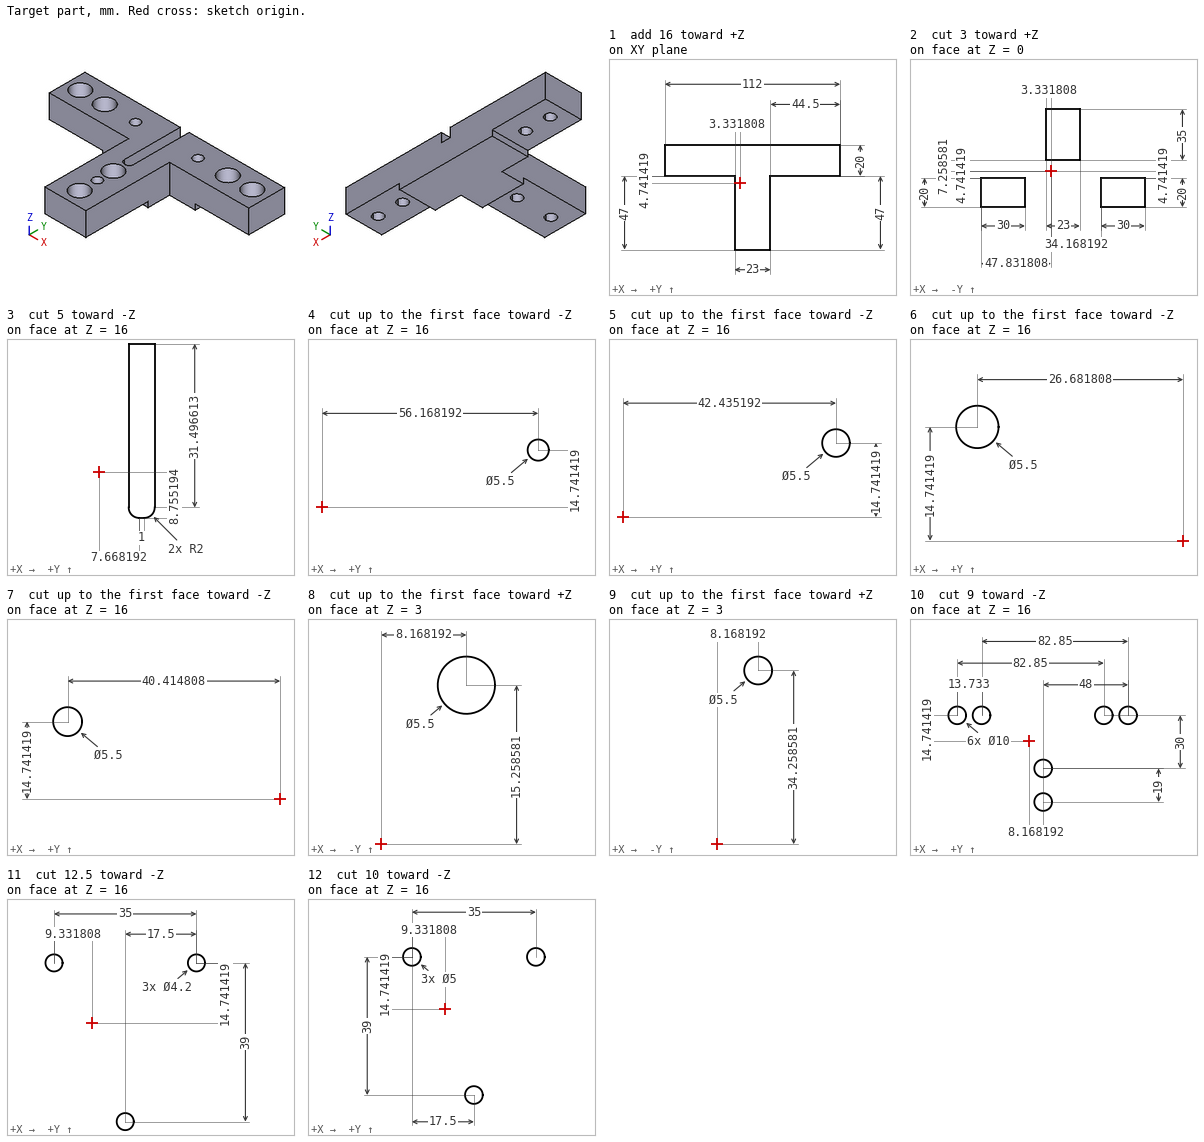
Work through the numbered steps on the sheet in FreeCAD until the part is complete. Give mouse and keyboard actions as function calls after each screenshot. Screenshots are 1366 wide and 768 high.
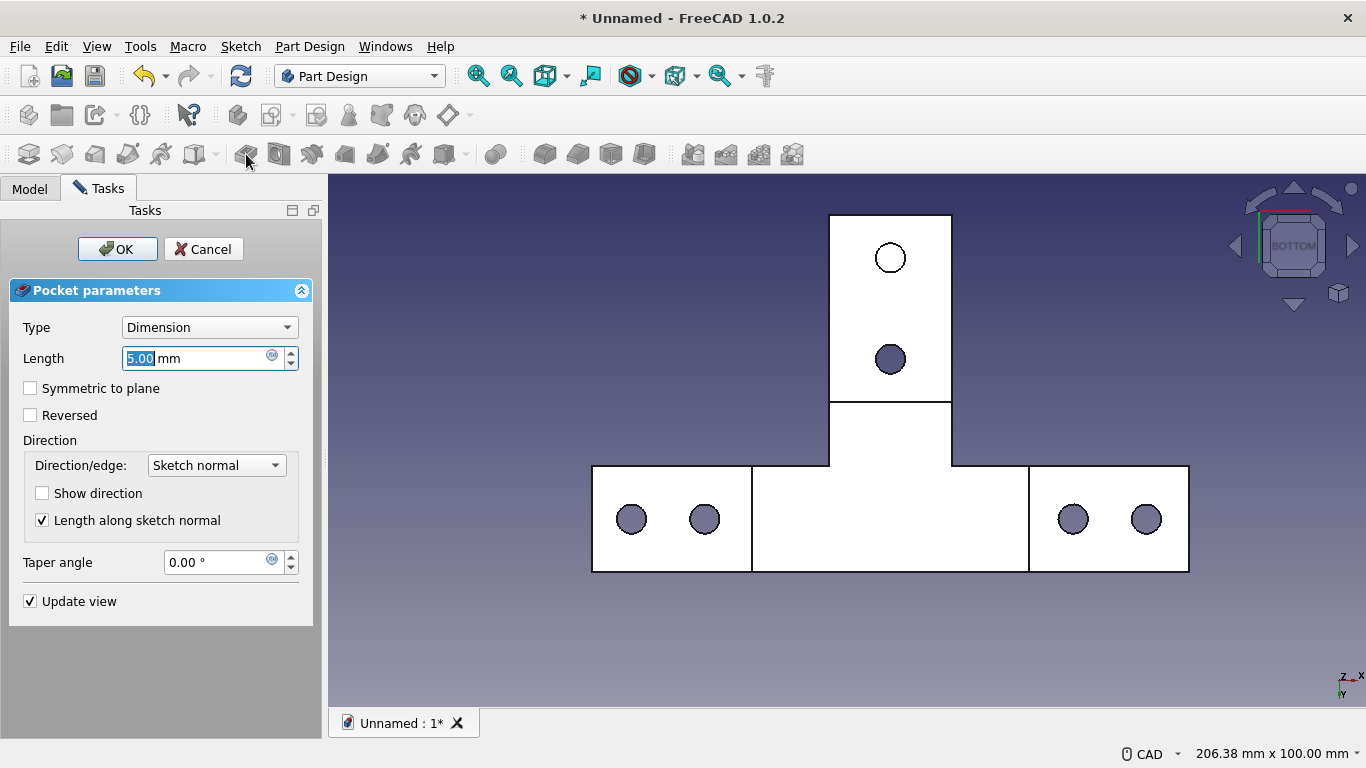
click(210, 328)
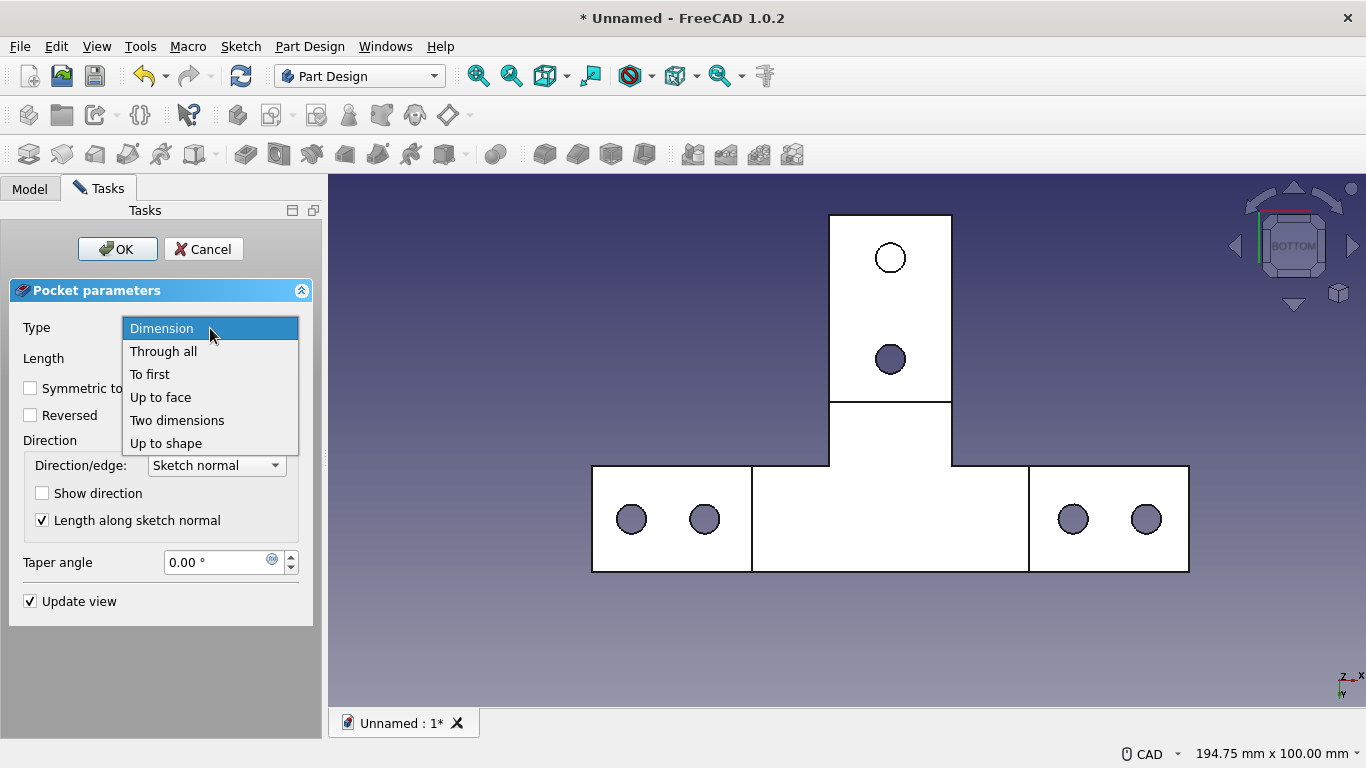
click(208, 374)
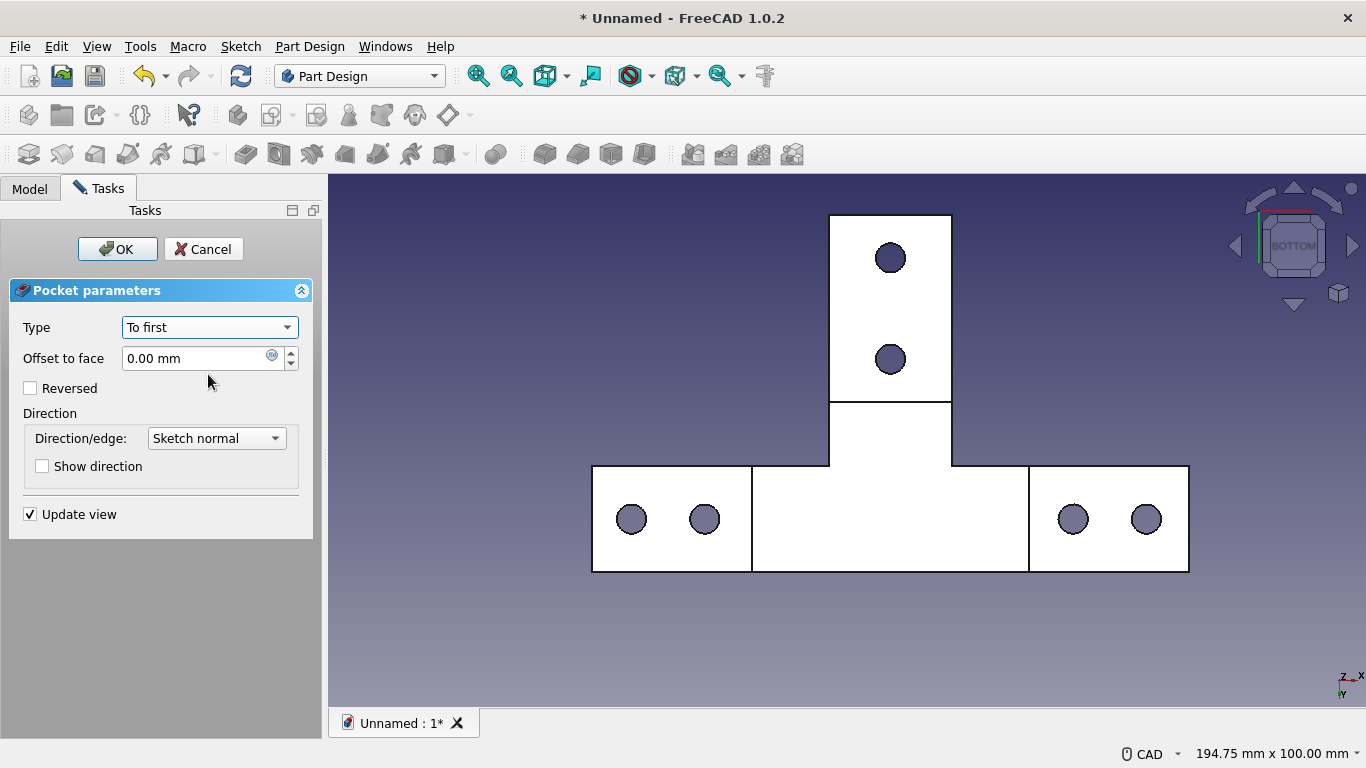
click(118, 249)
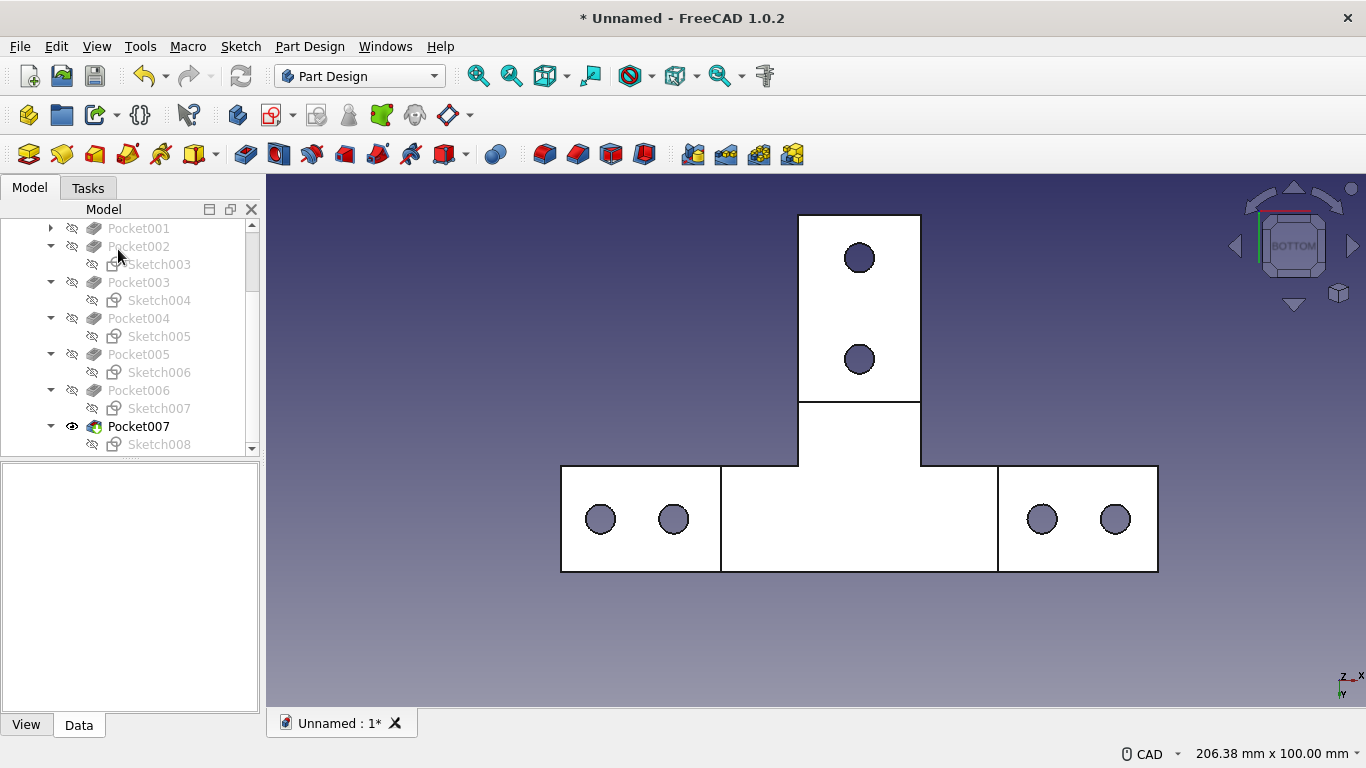
key(0)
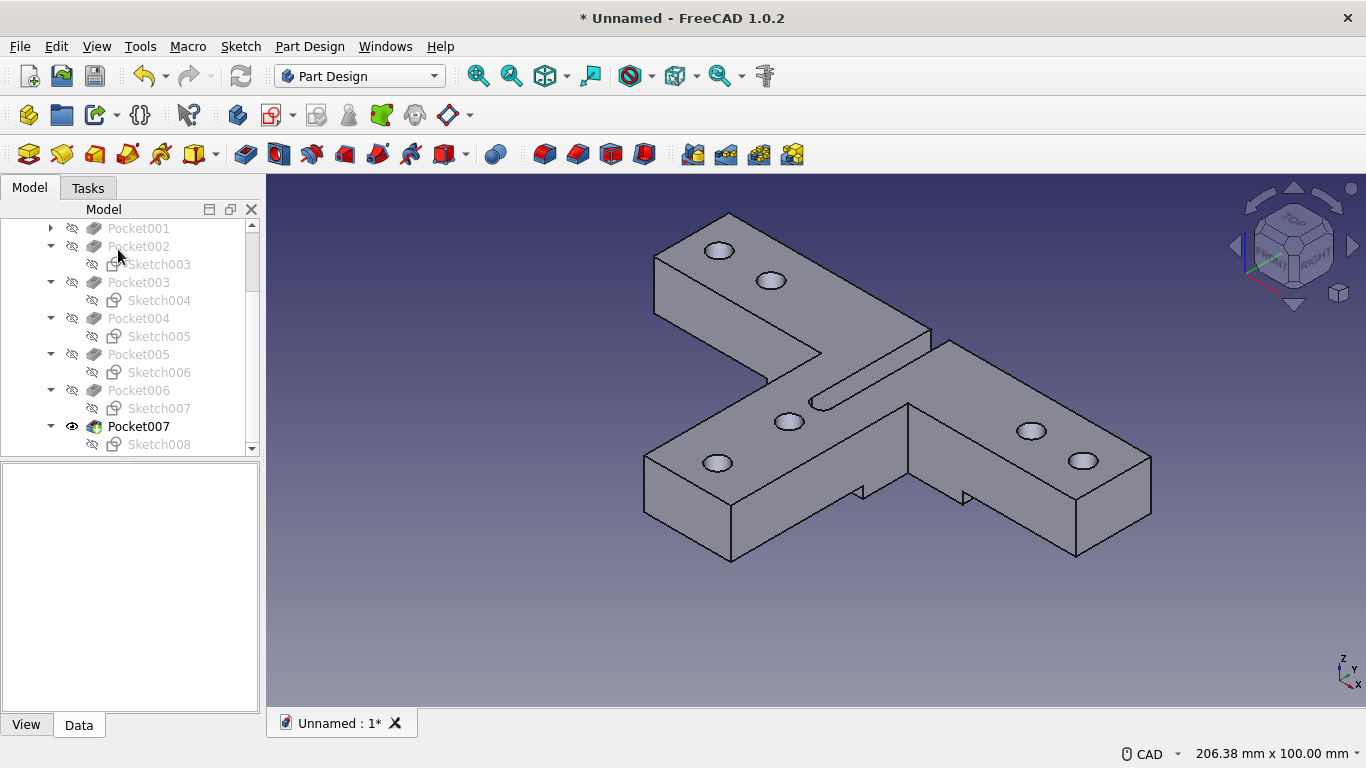
click(826, 330)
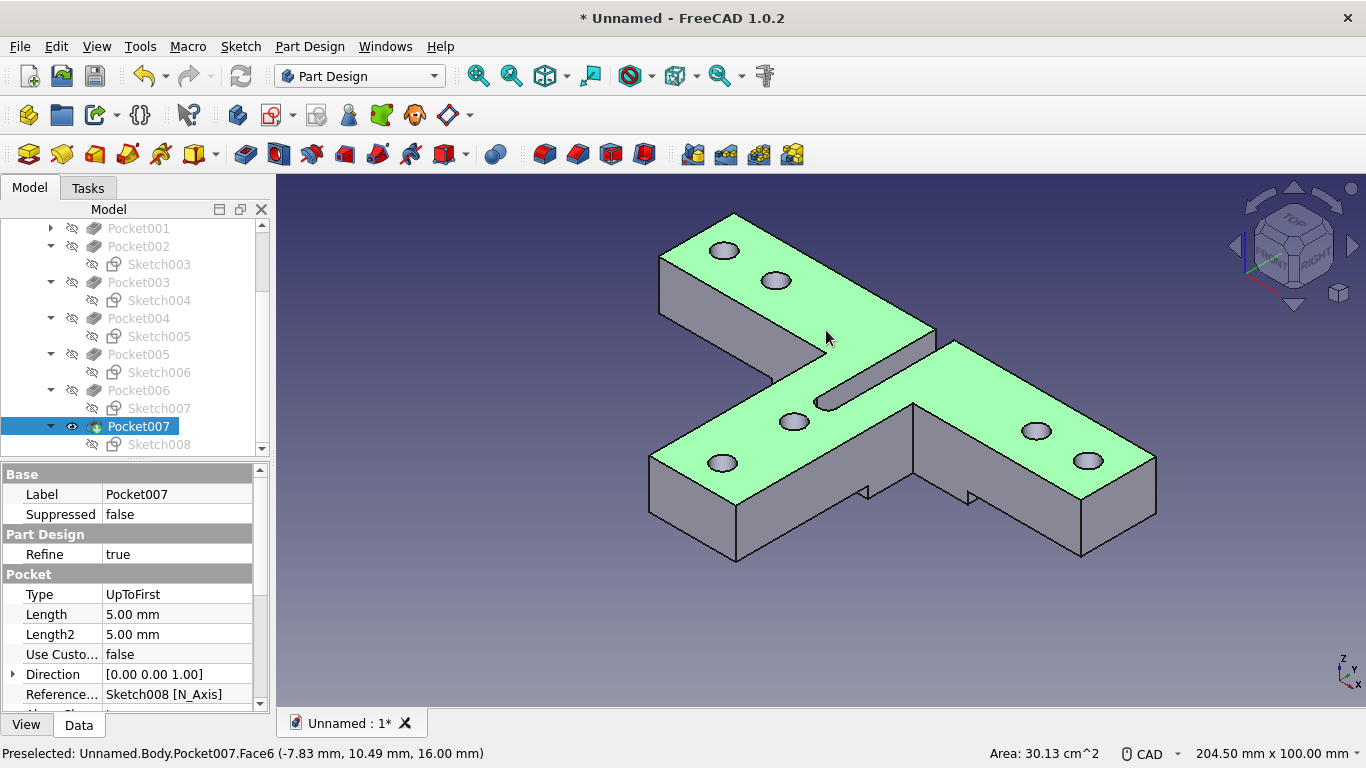
click(270, 116)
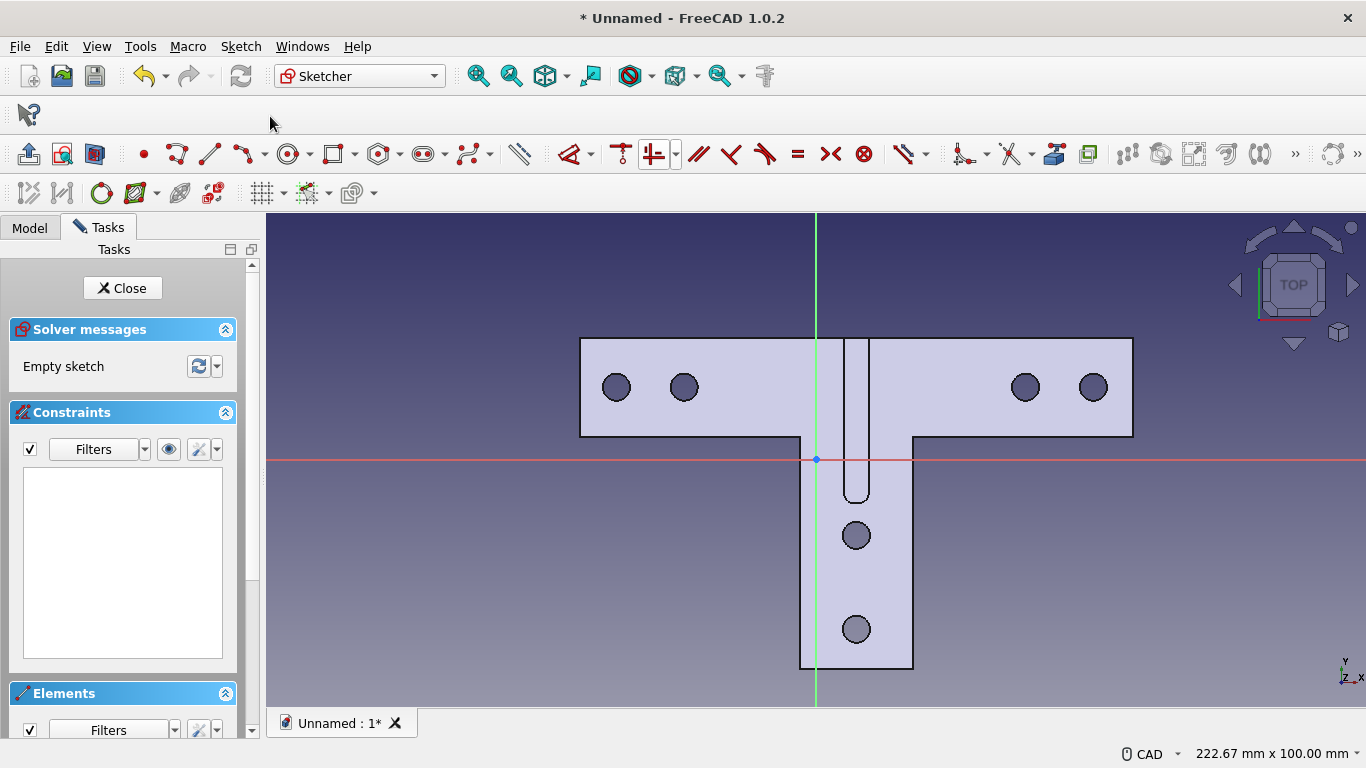
key(g)
key(c)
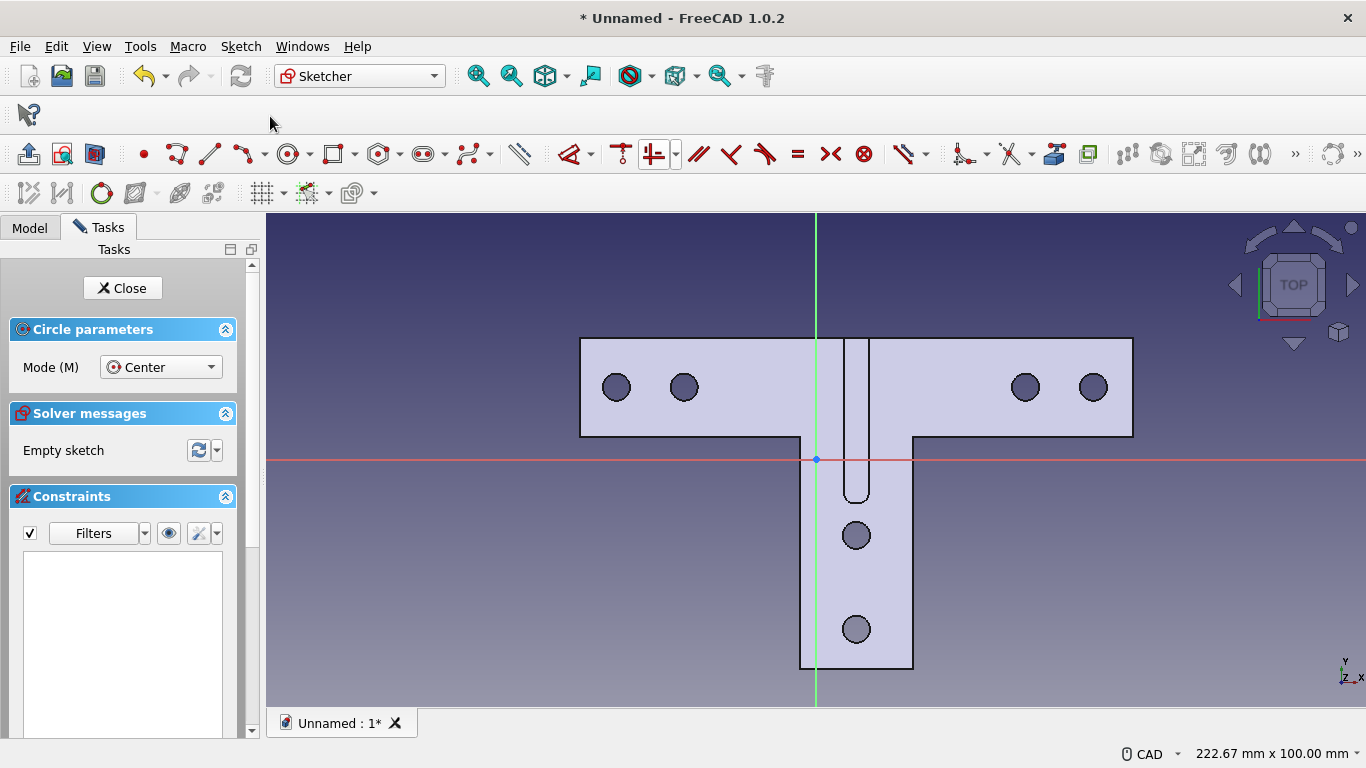
click(616, 387)
move(634, 370)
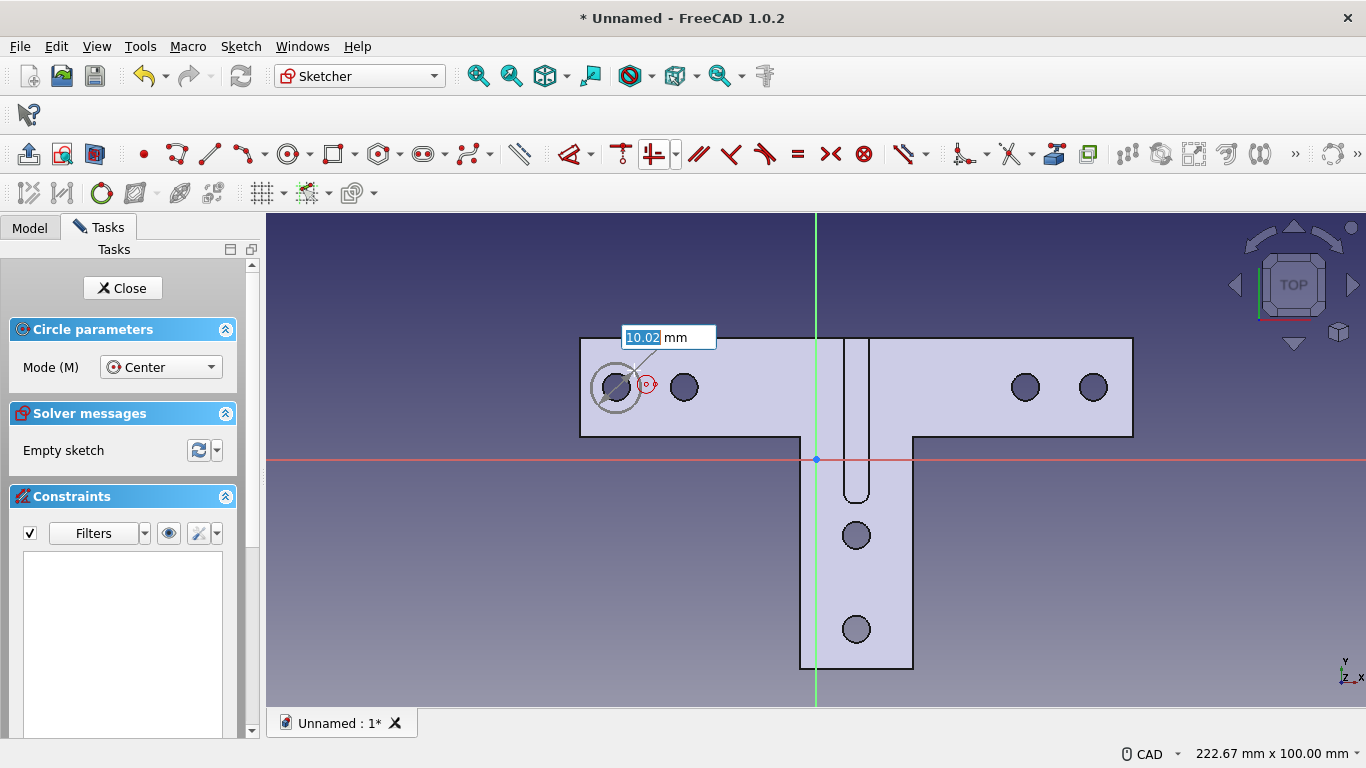
text(10)
key(Return)